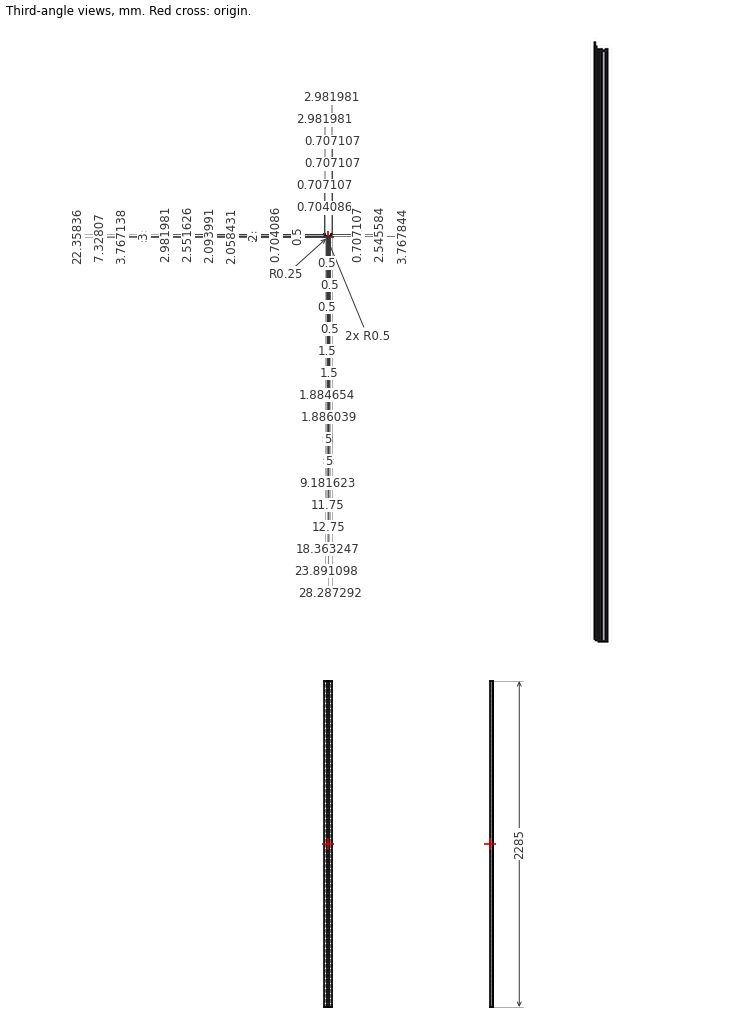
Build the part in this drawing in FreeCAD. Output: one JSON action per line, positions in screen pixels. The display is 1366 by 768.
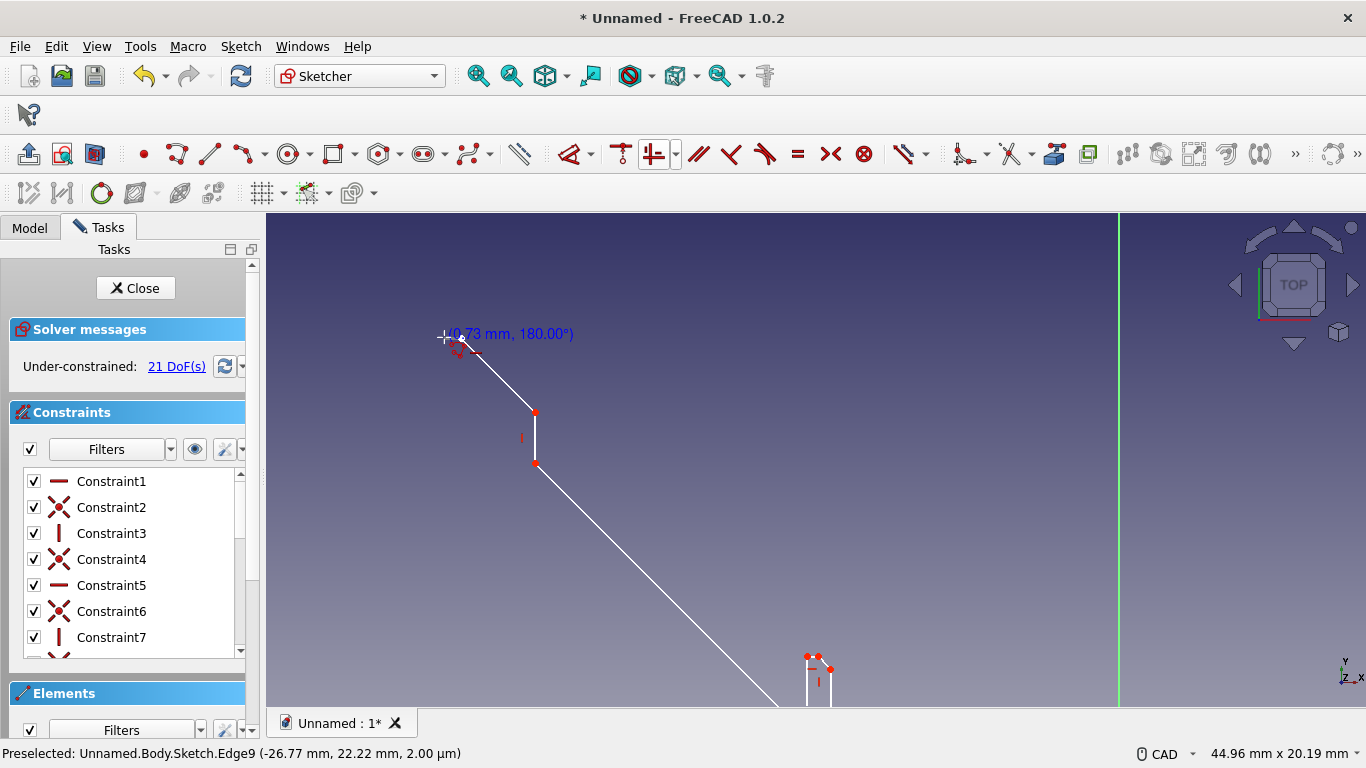
{"action": "left_click", "coordinate": [444, 337]}
{"action": "left_click", "coordinate": [427, 355]}
{"action": "left_click", "coordinate": [427, 417]}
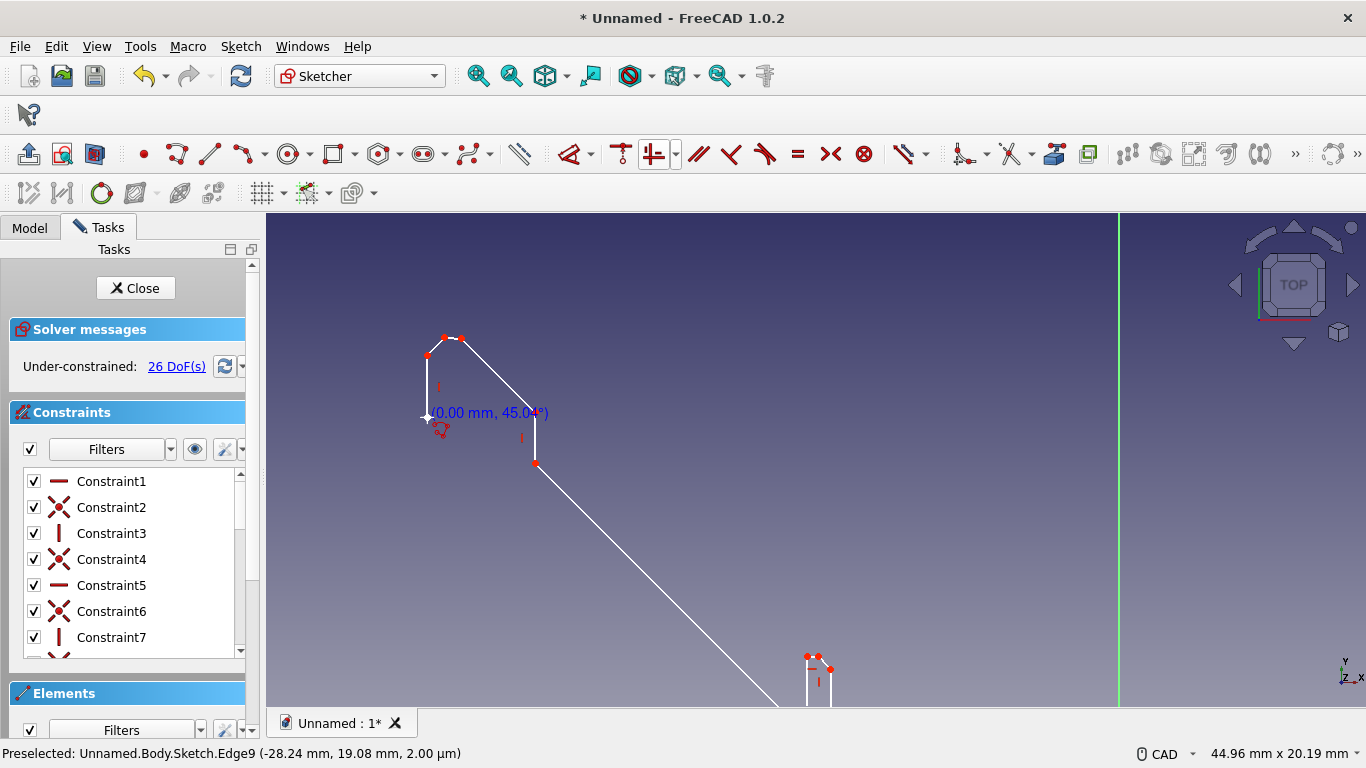
{"action": "scroll", "coordinate": [444, 337], "scroll_direction": "down", "scroll_amount": 4}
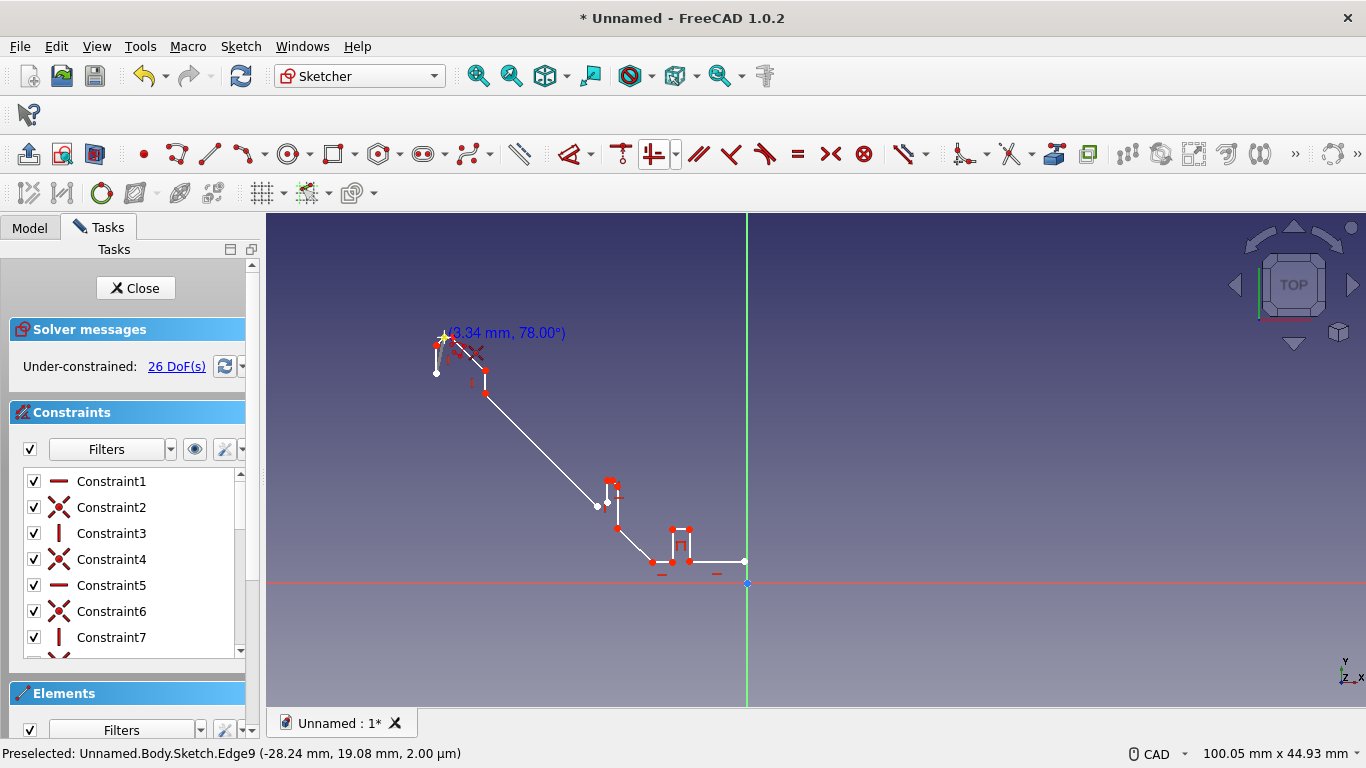
{"action": "left_click", "coordinate": [646, 583]}
{"action": "left_click", "coordinate": [848, 574]}
{"action": "left_click", "coordinate": [1058, 373]}
{"action": "left_click", "coordinate": [1058, 345]}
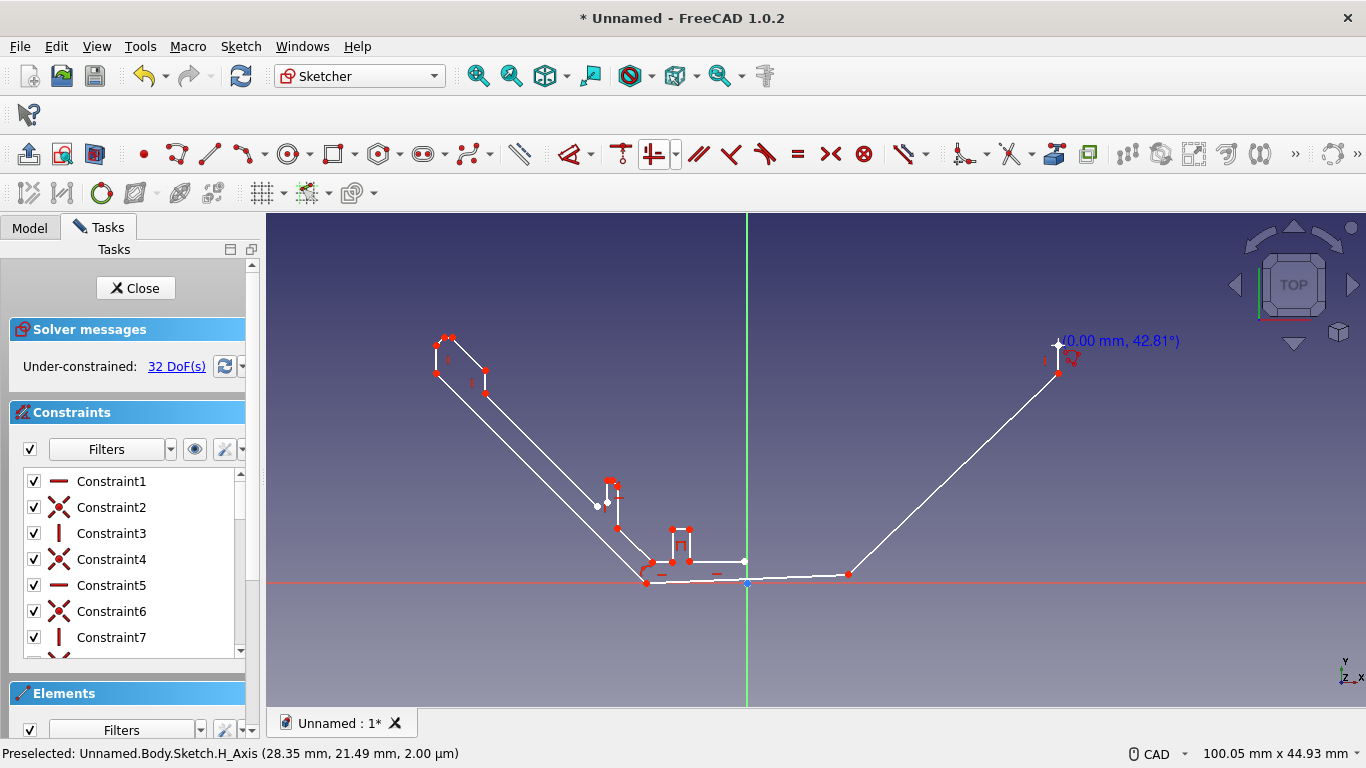
{"action": "scroll", "coordinate": [1051, 337], "scroll_direction": "up", "scroll_amount": 2}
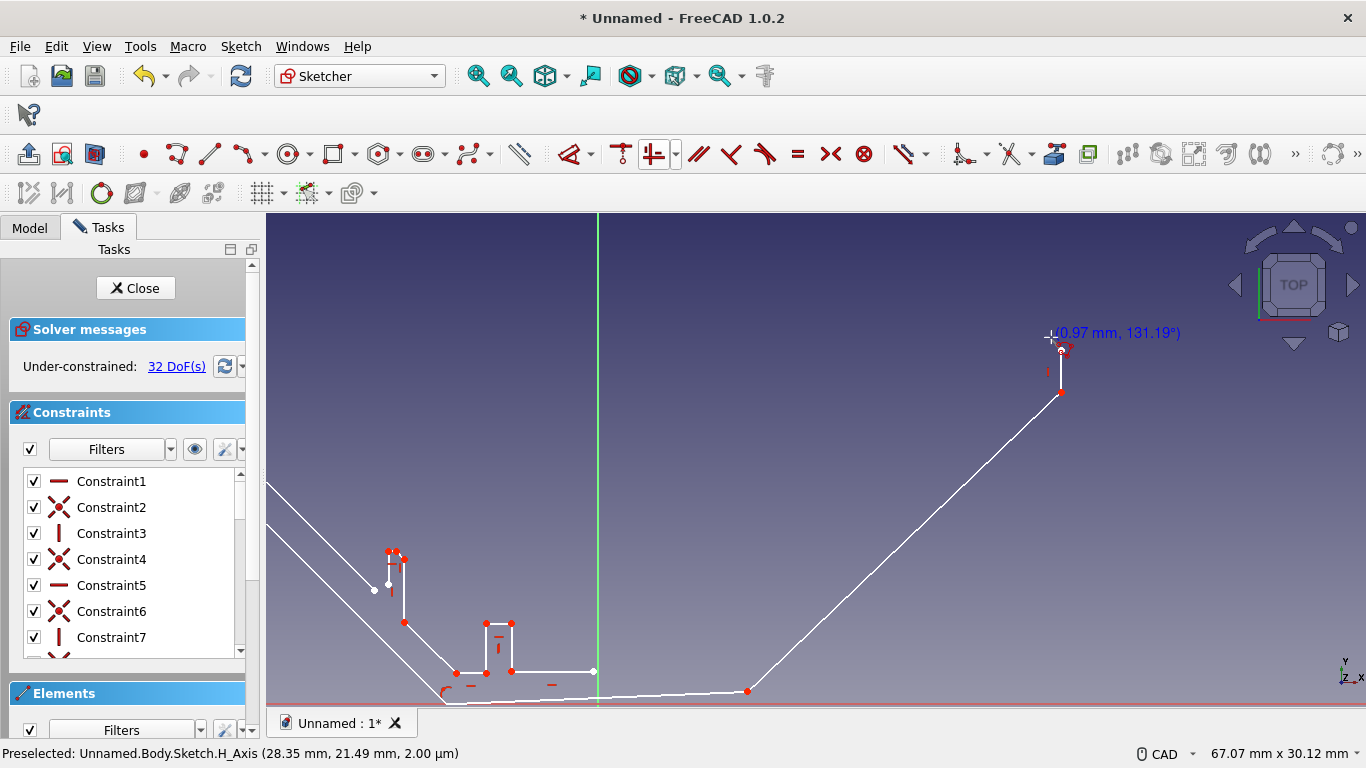
{"action": "left_click", "coordinate": [1050, 338]}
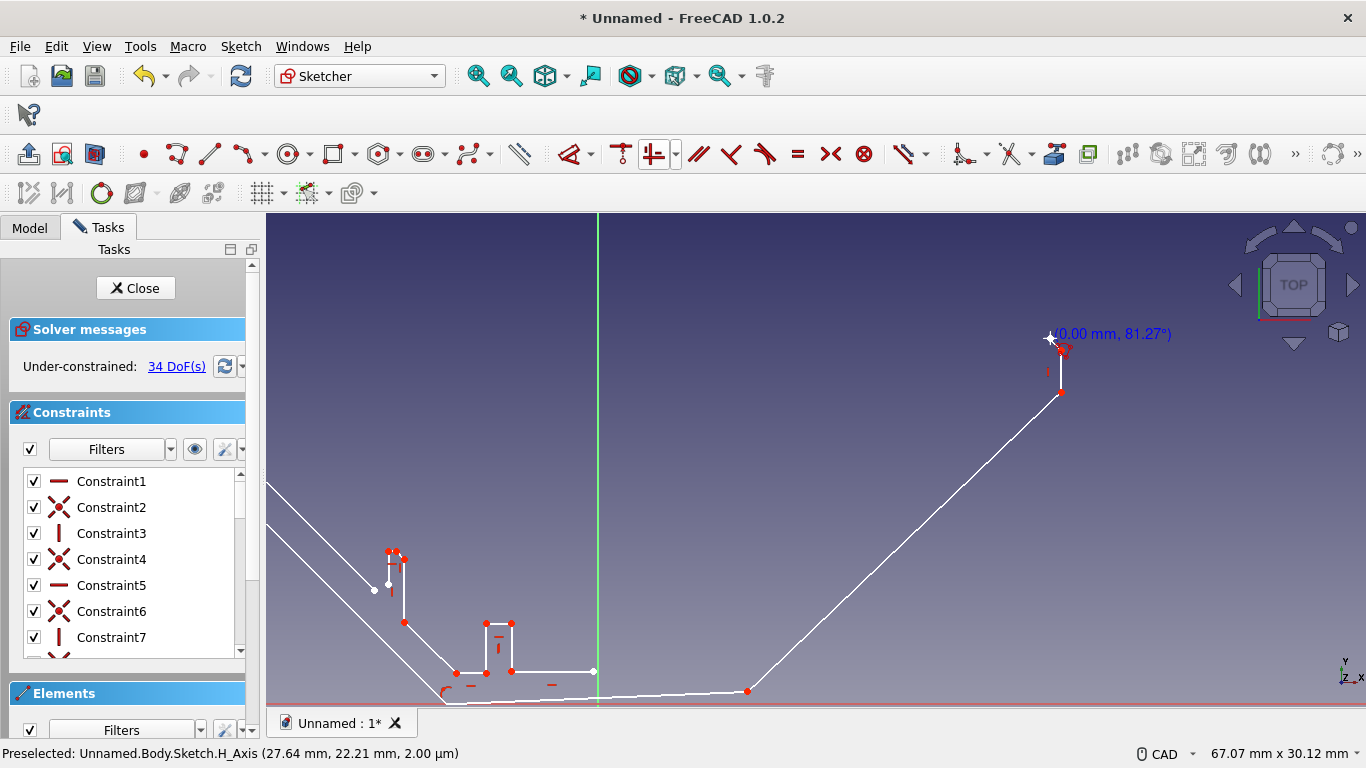
{"action": "scroll", "coordinate": [1038, 338], "scroll_direction": "up", "scroll_amount": 2}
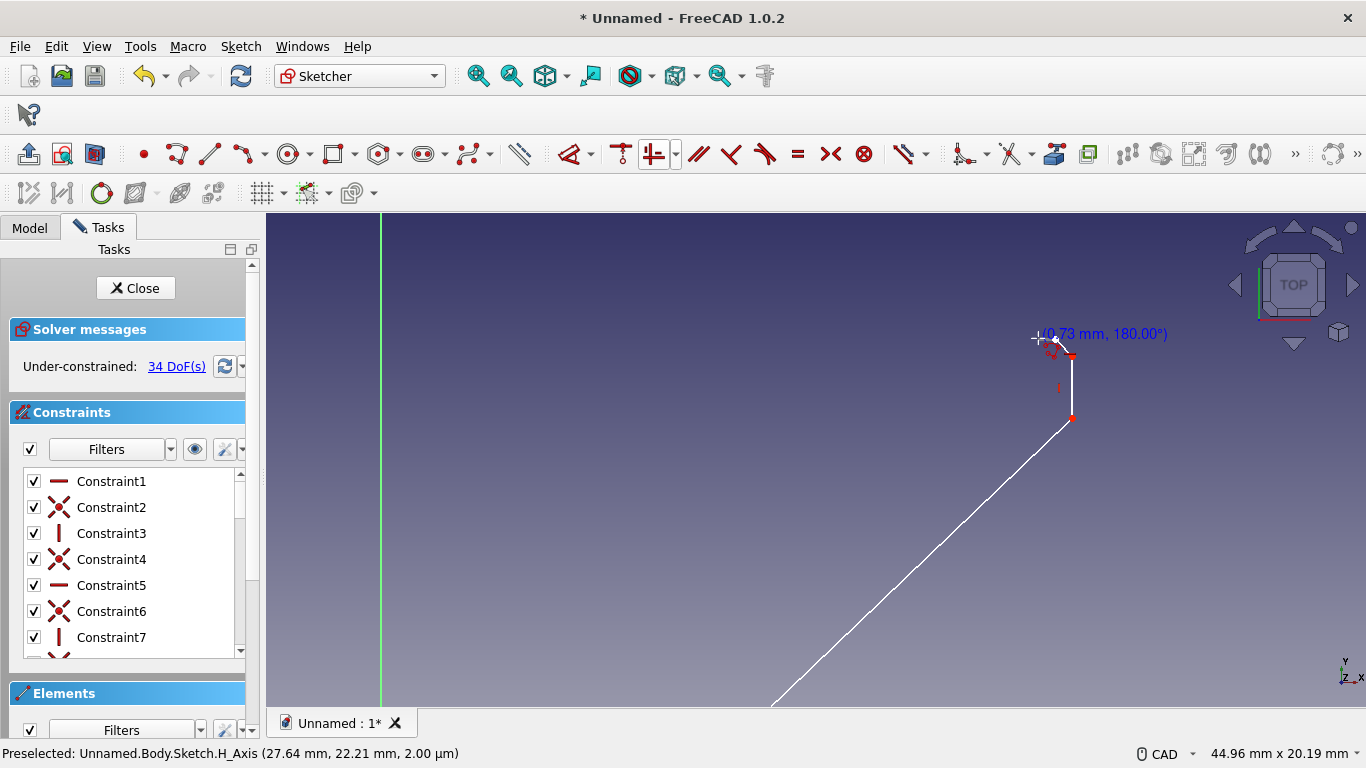
{"action": "left_click", "coordinate": [1038, 338]}
{"action": "left_click", "coordinate": [965, 410]}
{"action": "left_click", "coordinate": [965, 462]}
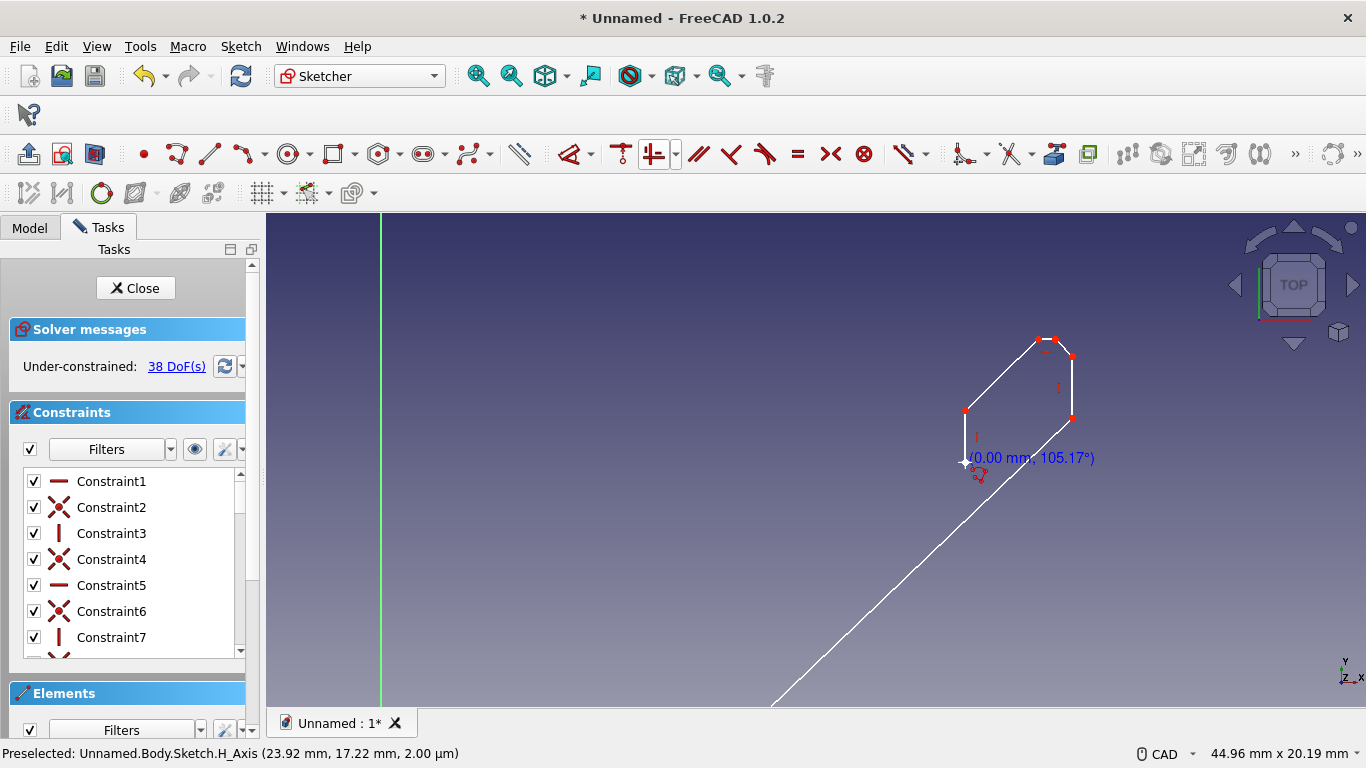
{"action": "scroll", "coordinate": [1047, 337], "scroll_direction": "down", "scroll_amount": 4}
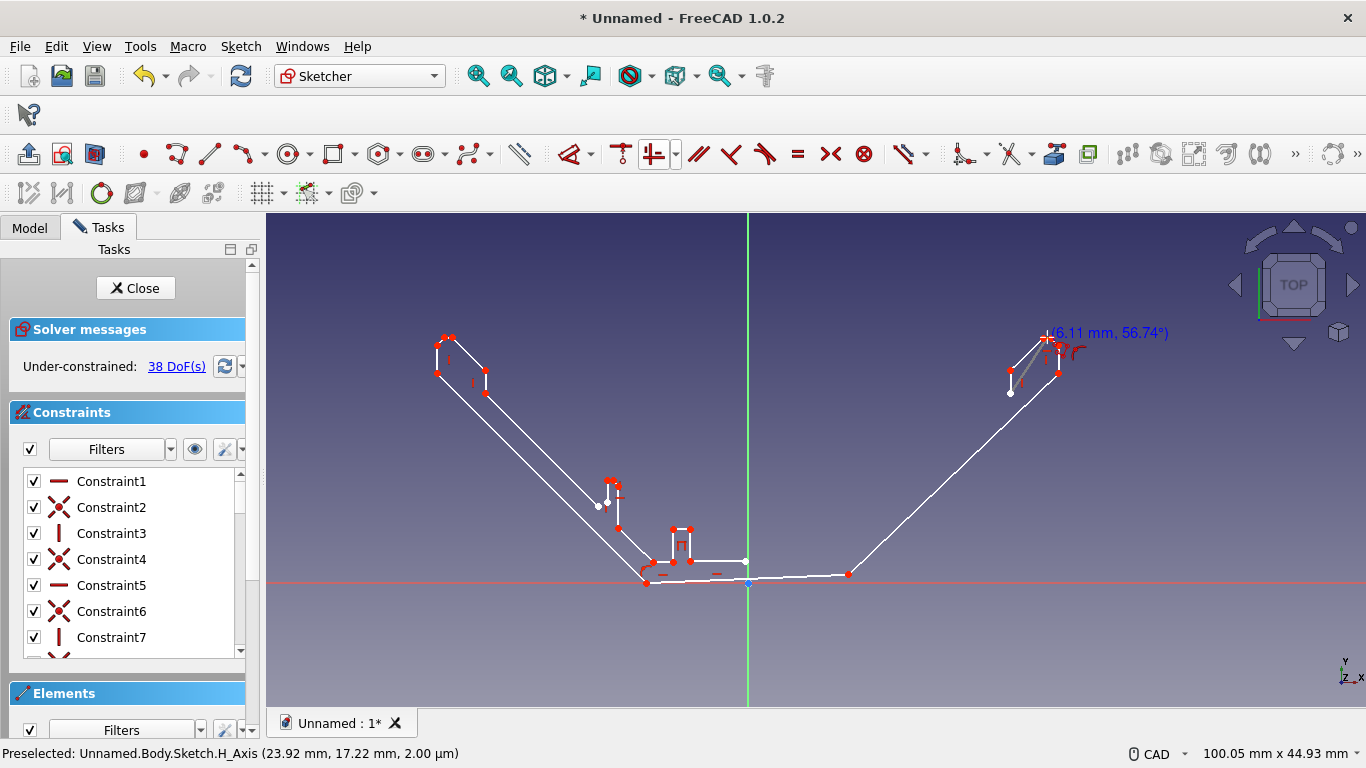
{"action": "left_click", "coordinate": [898, 506]}
{"action": "right_click", "coordinate": [898, 506]}